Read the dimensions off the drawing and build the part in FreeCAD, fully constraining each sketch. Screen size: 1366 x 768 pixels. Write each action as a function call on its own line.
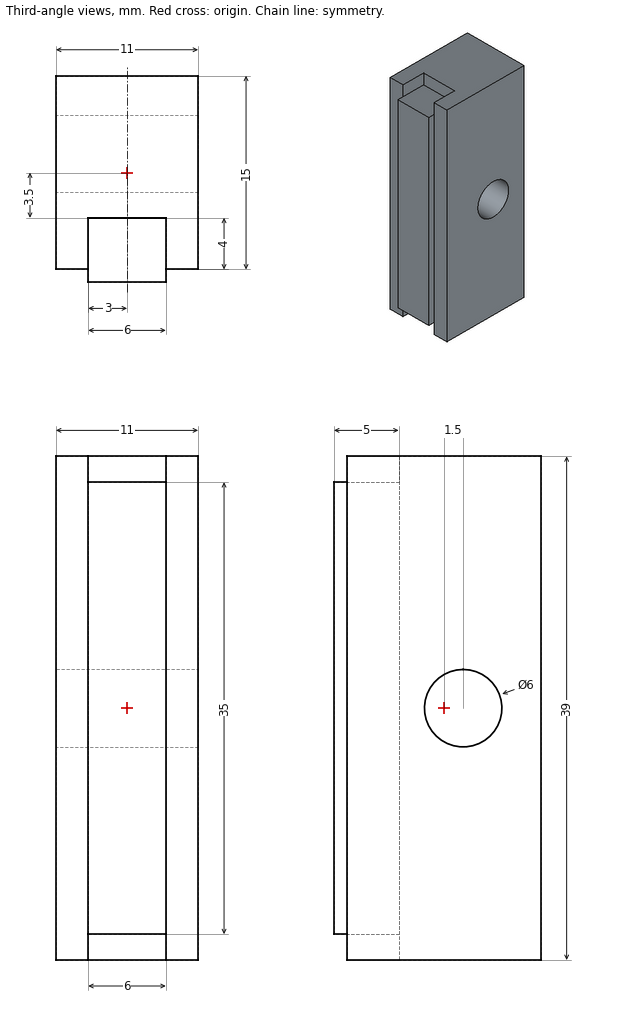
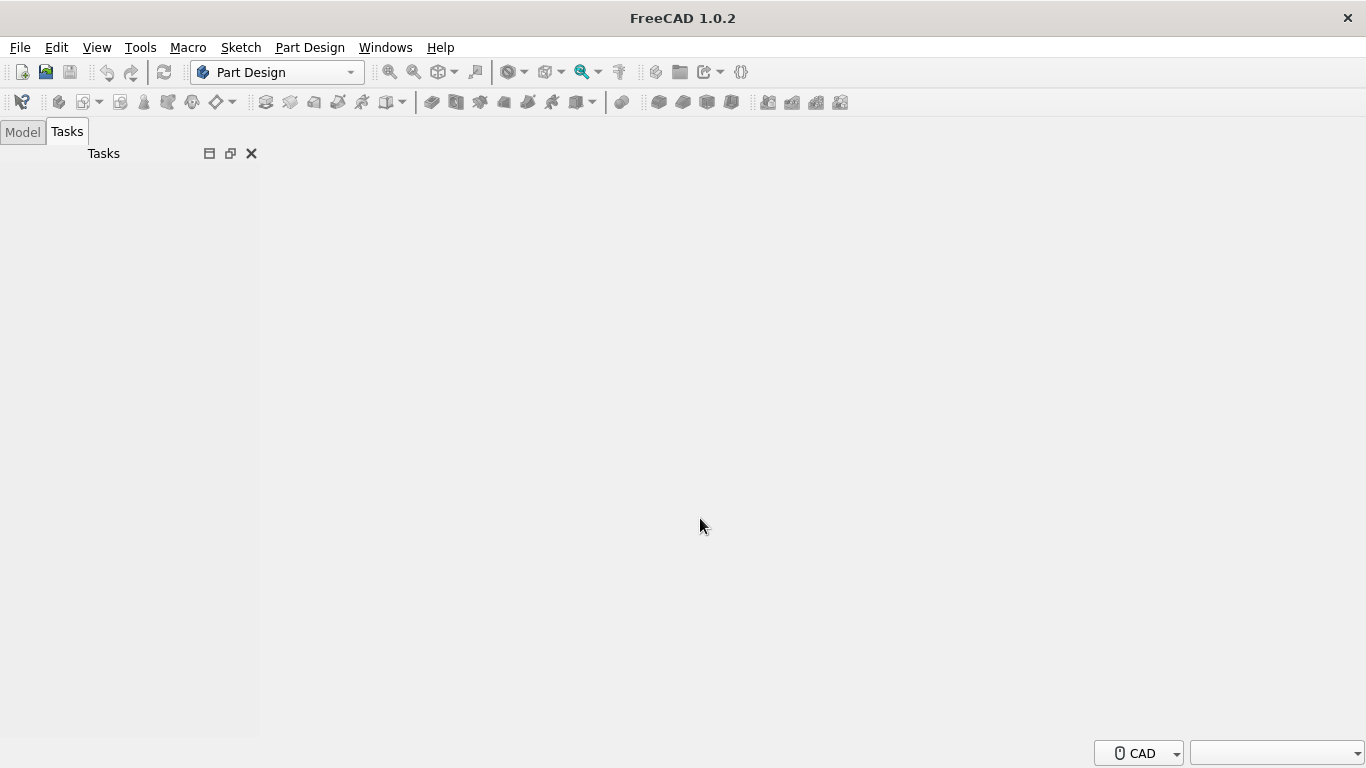
click(22, 72)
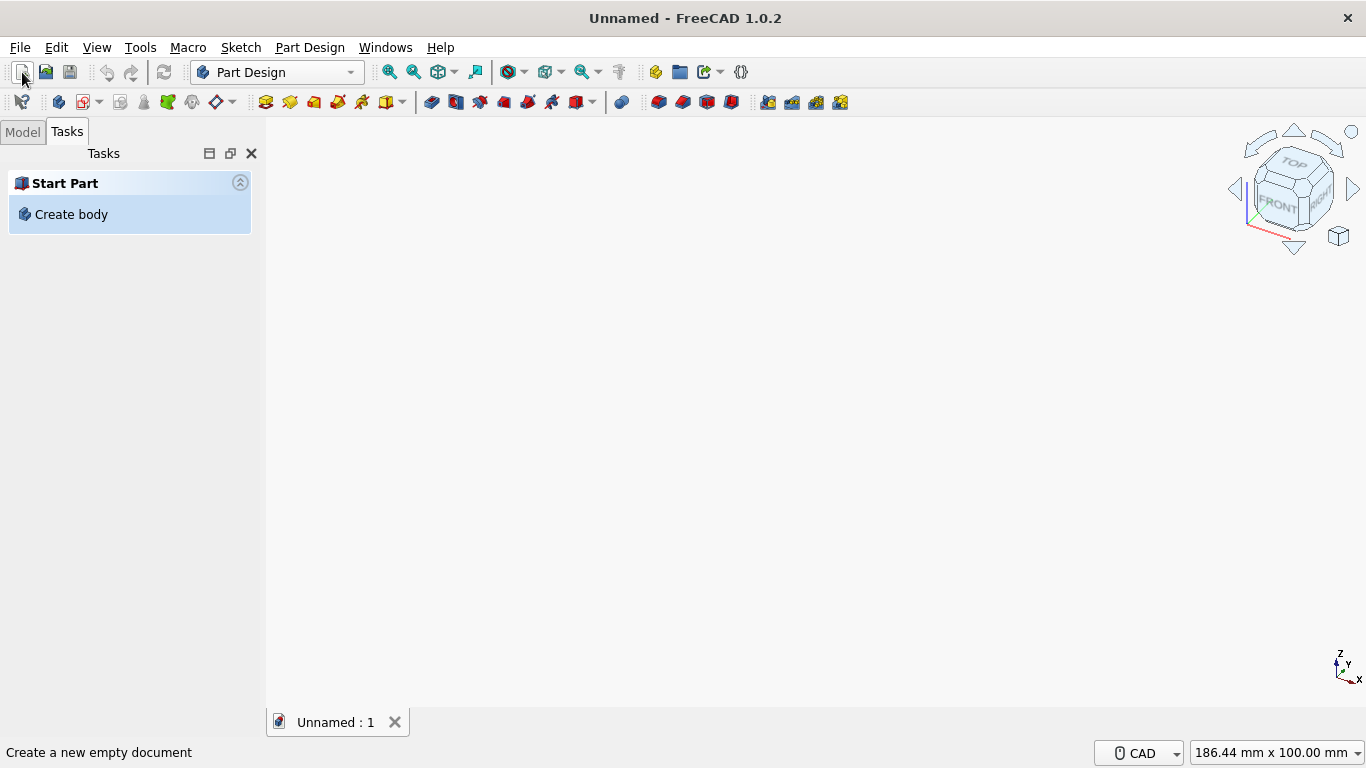
click(84, 102)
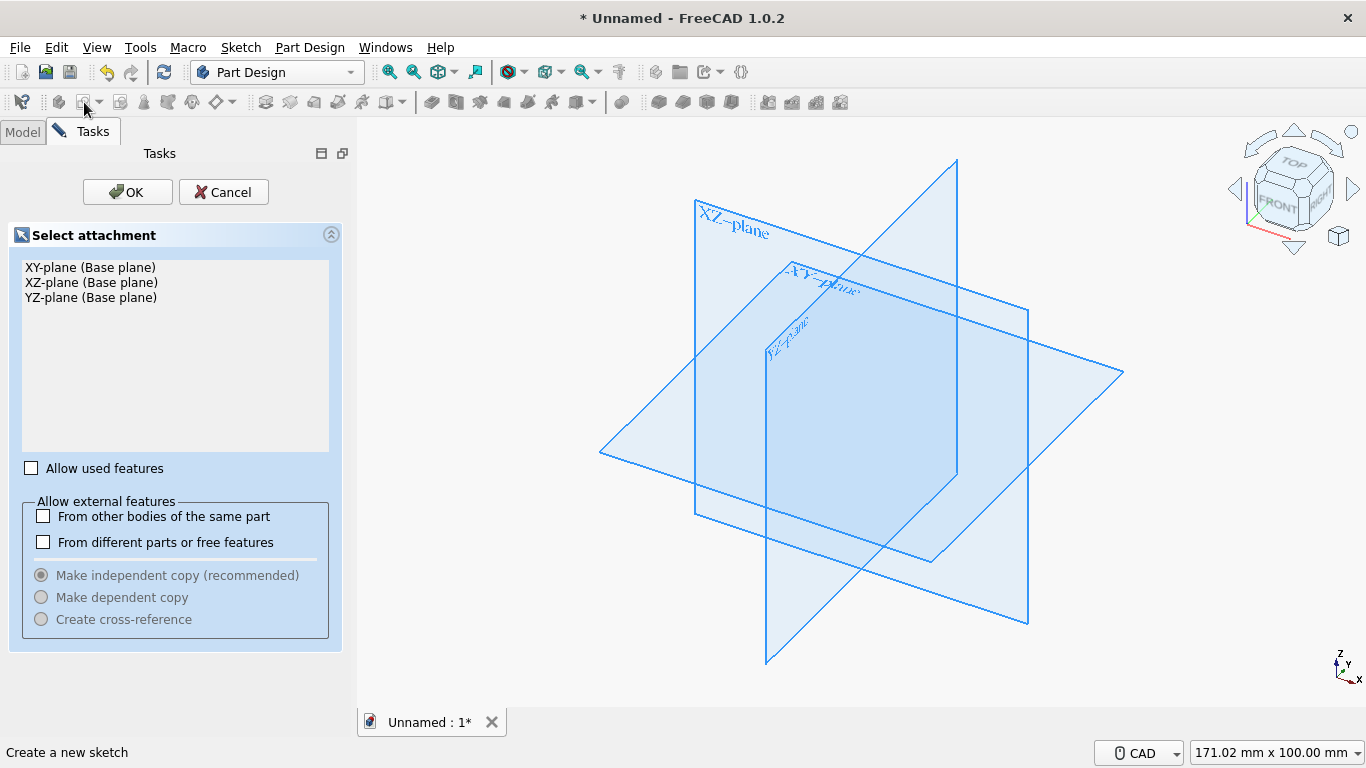
click(82, 268)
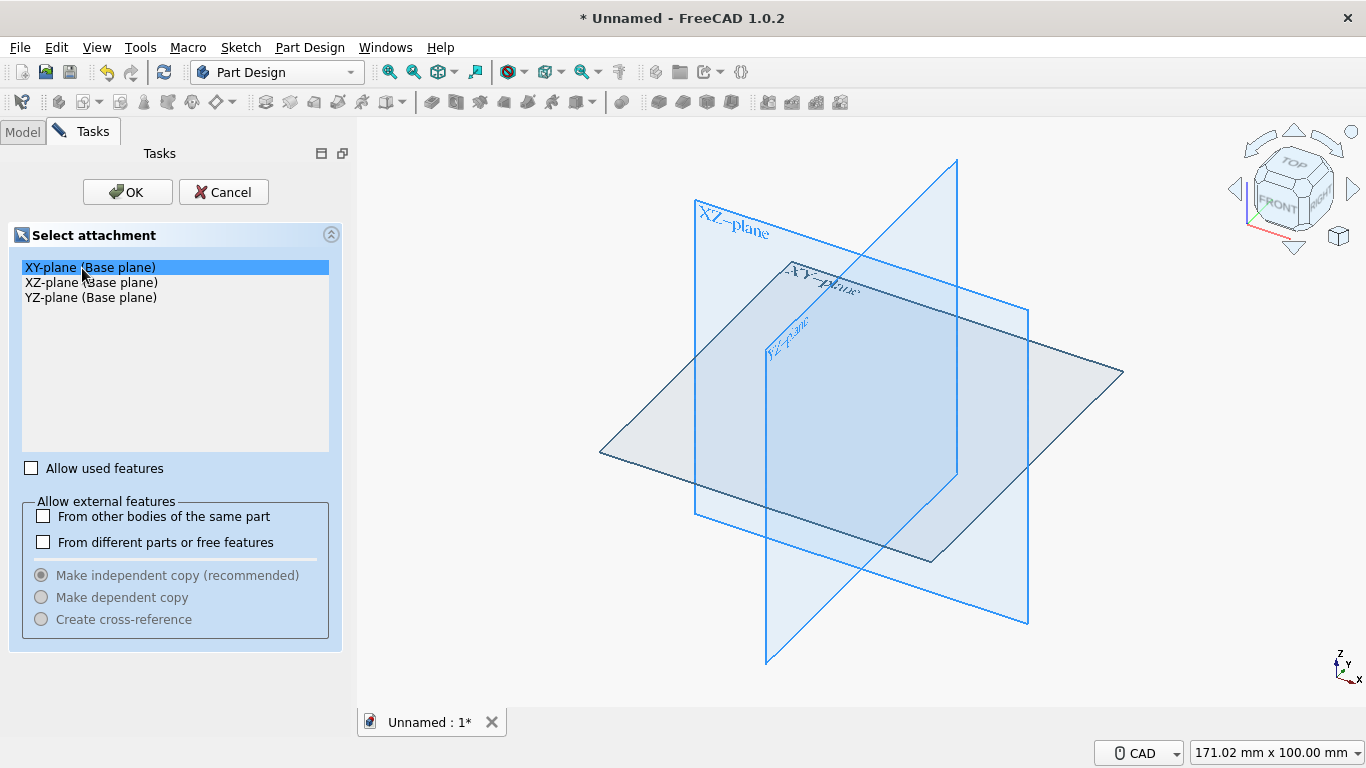
click(128, 192)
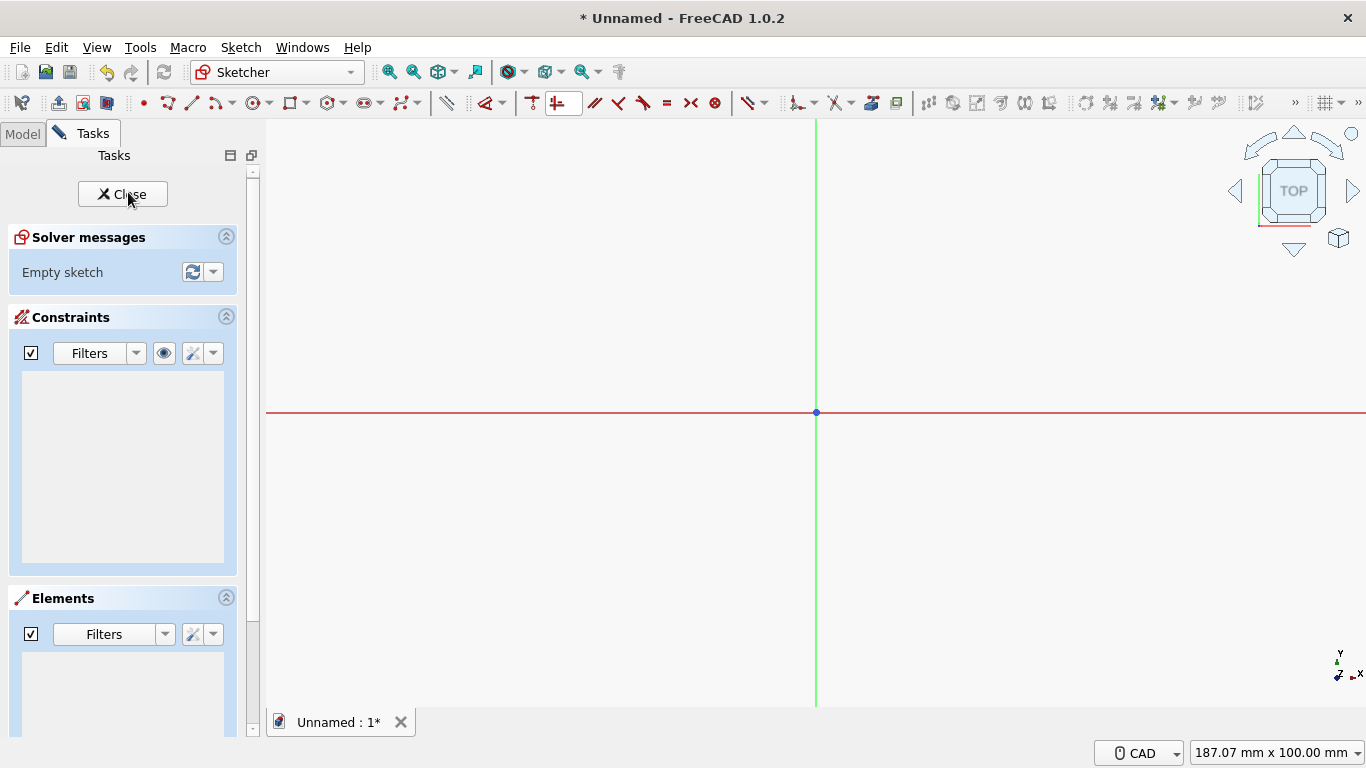
scroll(838, 413, up, 7)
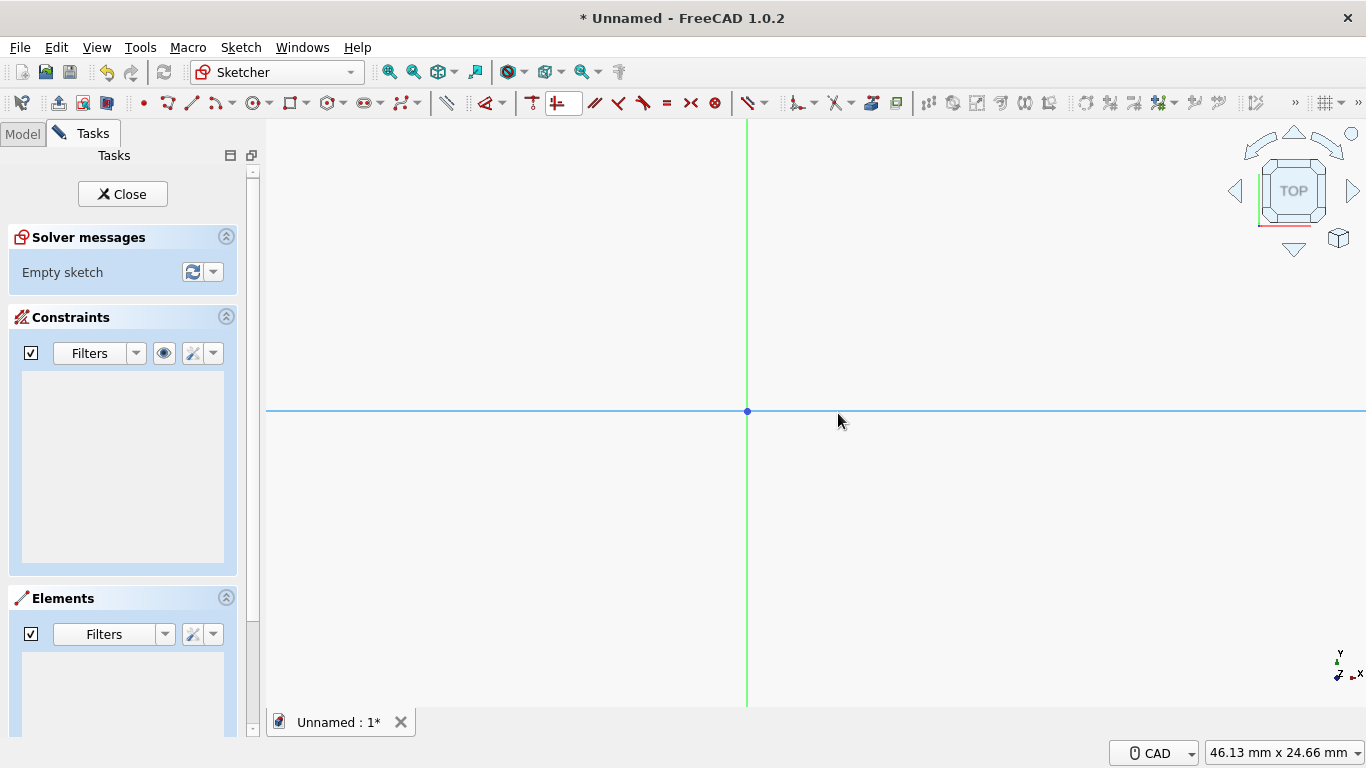
click(168, 104)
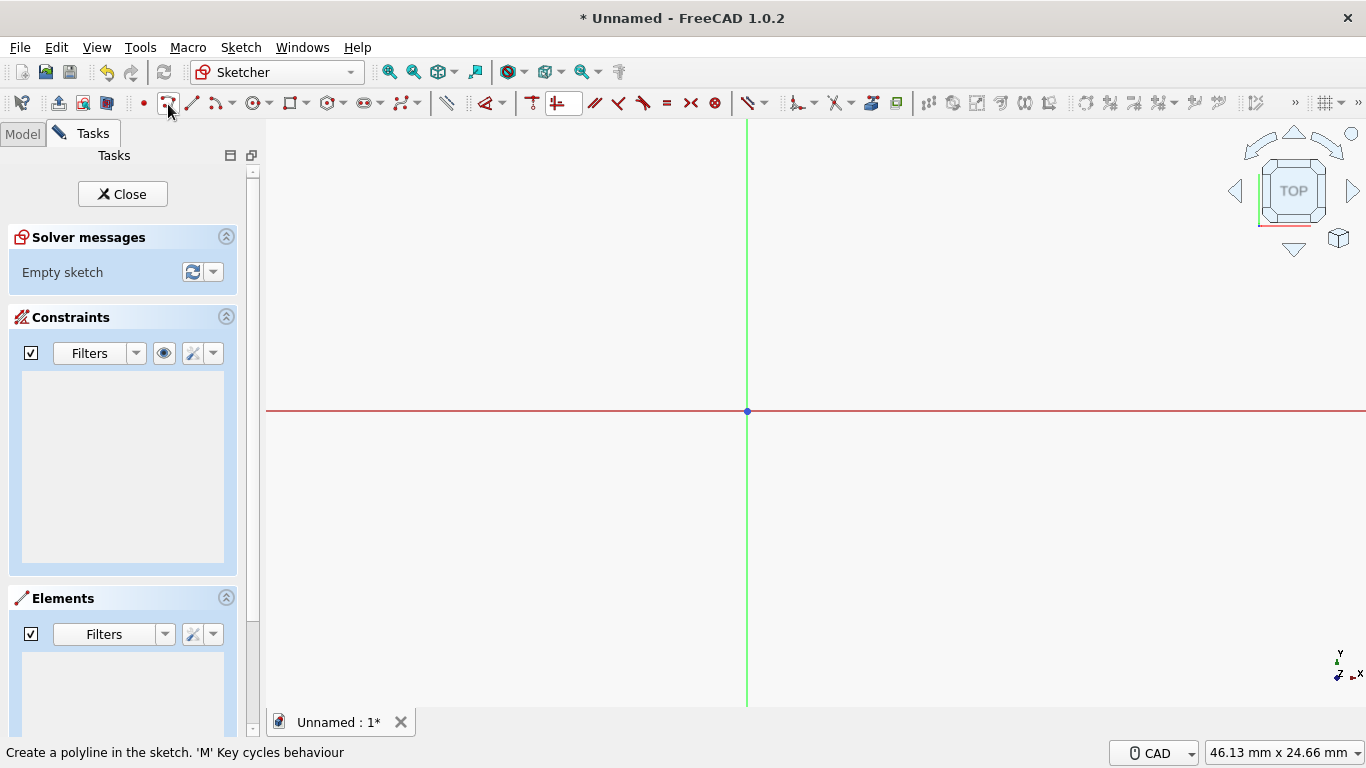
click(676, 495)
click(819, 495)
click(819, 590)
click(878, 590)
click(878, 233)
click(616, 233)
click(616, 590)
click(676, 590)
click(676, 496)
key(Escape)
key(Escape)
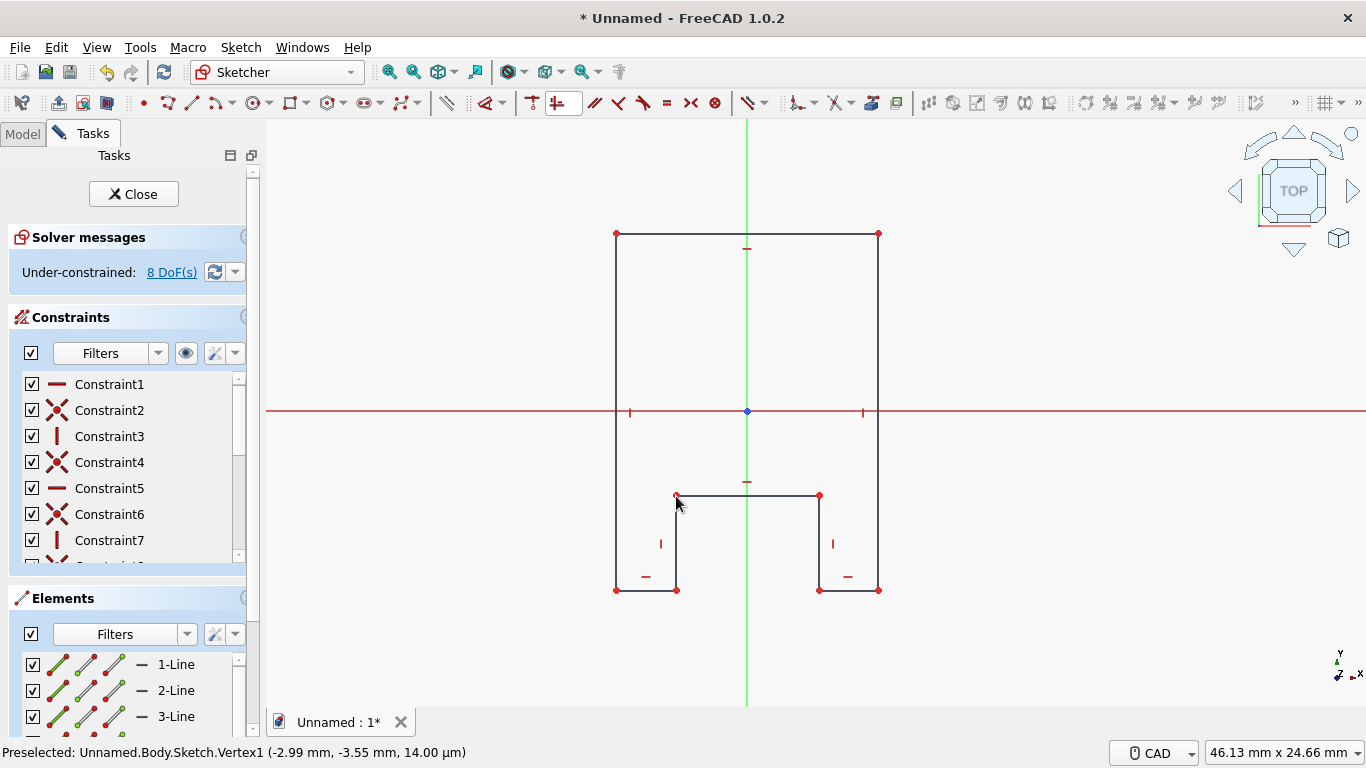
click(878, 591)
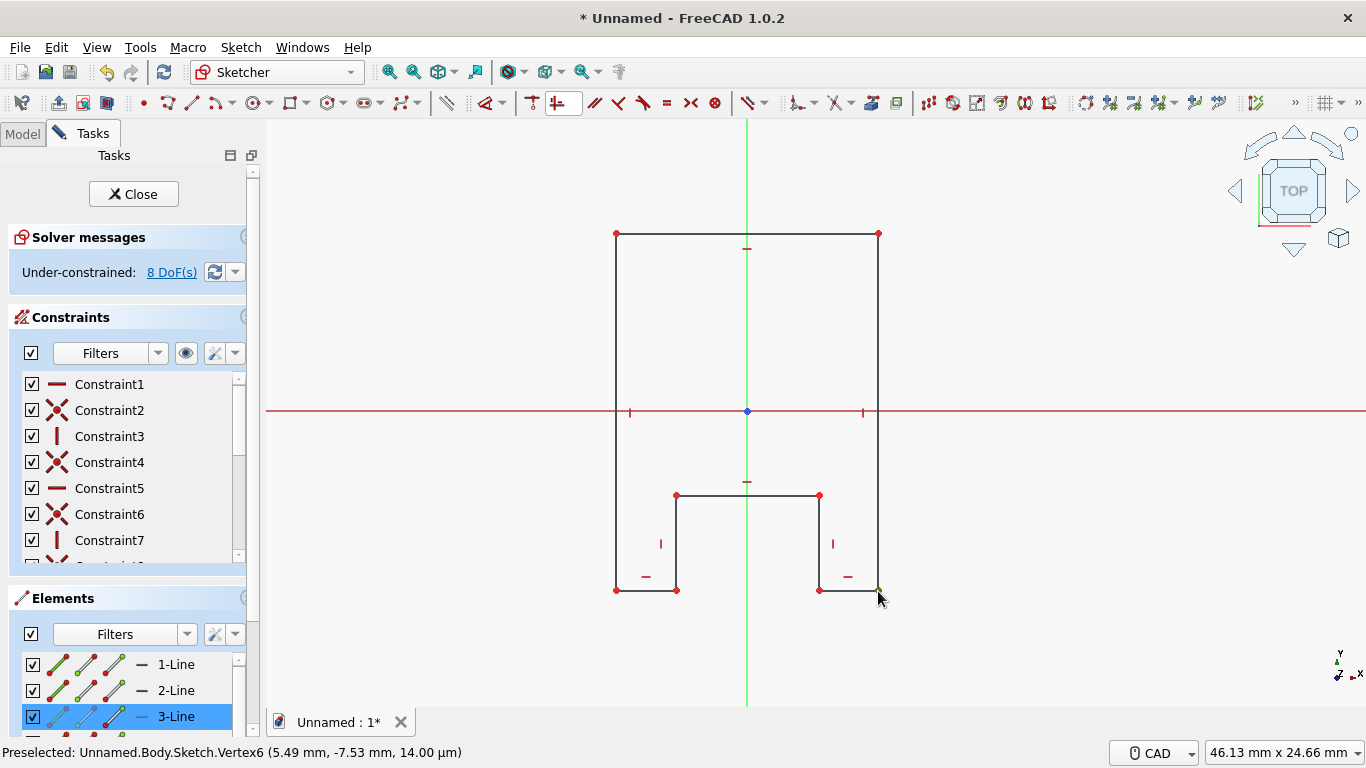
click(616, 591)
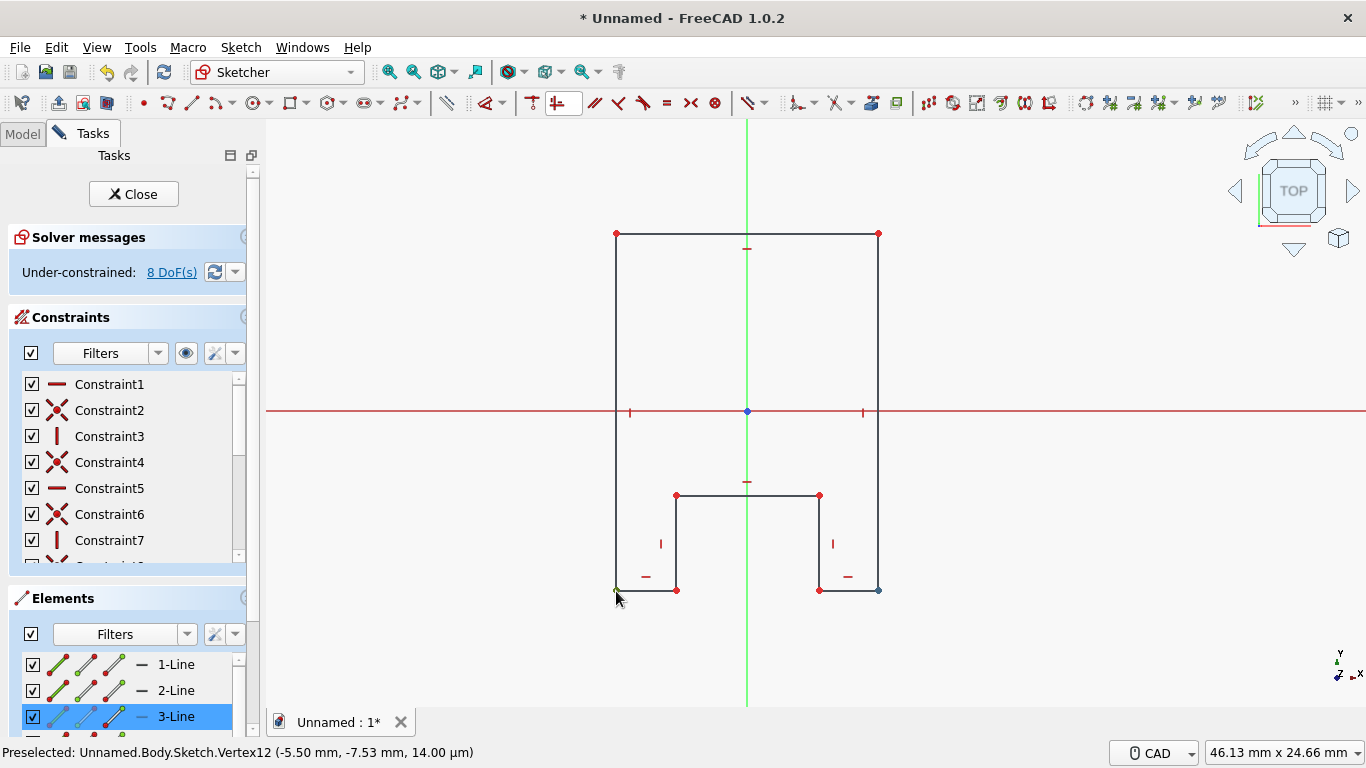
click(747, 641)